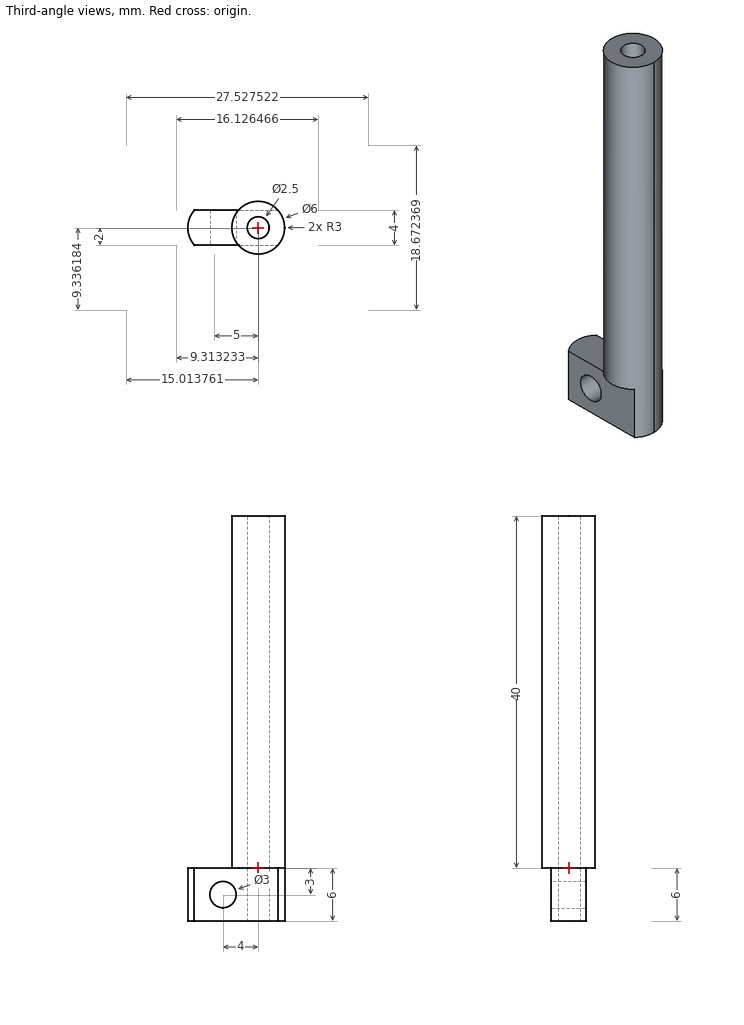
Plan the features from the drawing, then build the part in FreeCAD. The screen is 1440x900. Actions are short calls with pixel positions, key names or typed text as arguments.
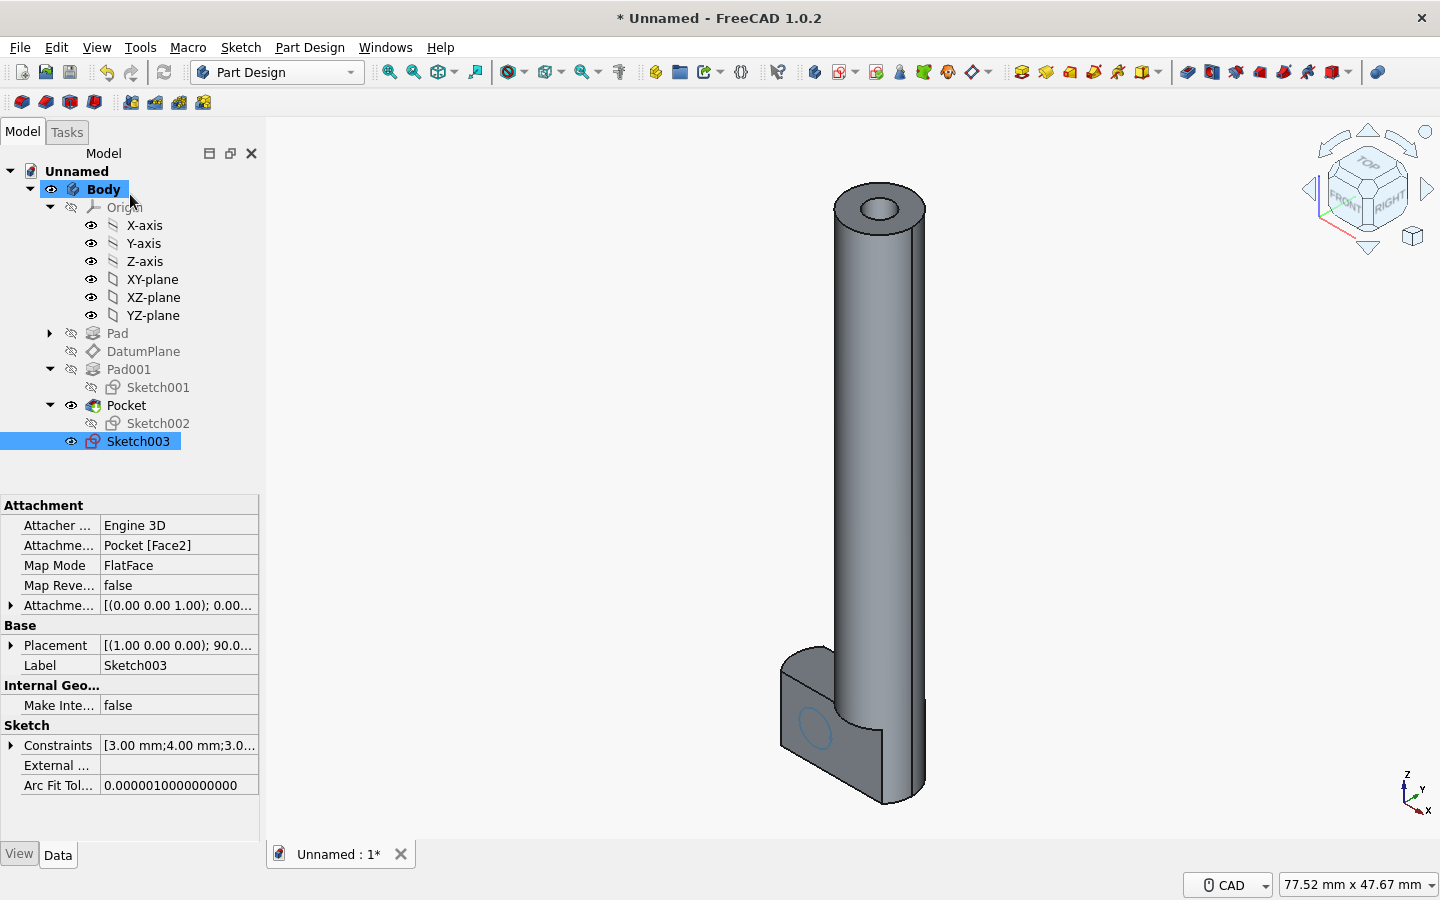
click(1188, 72)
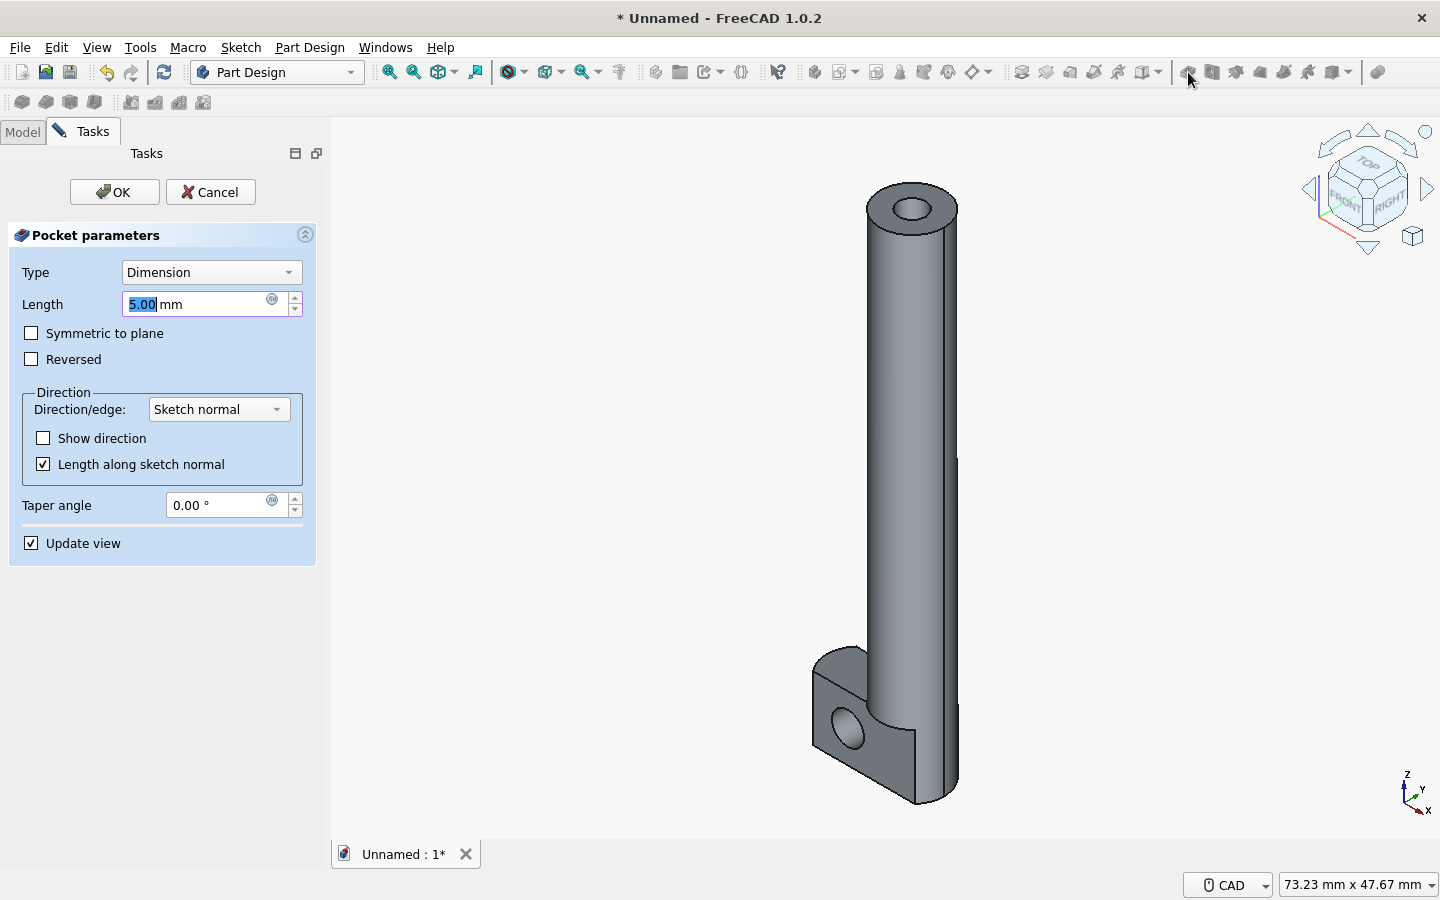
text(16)
key(Tab)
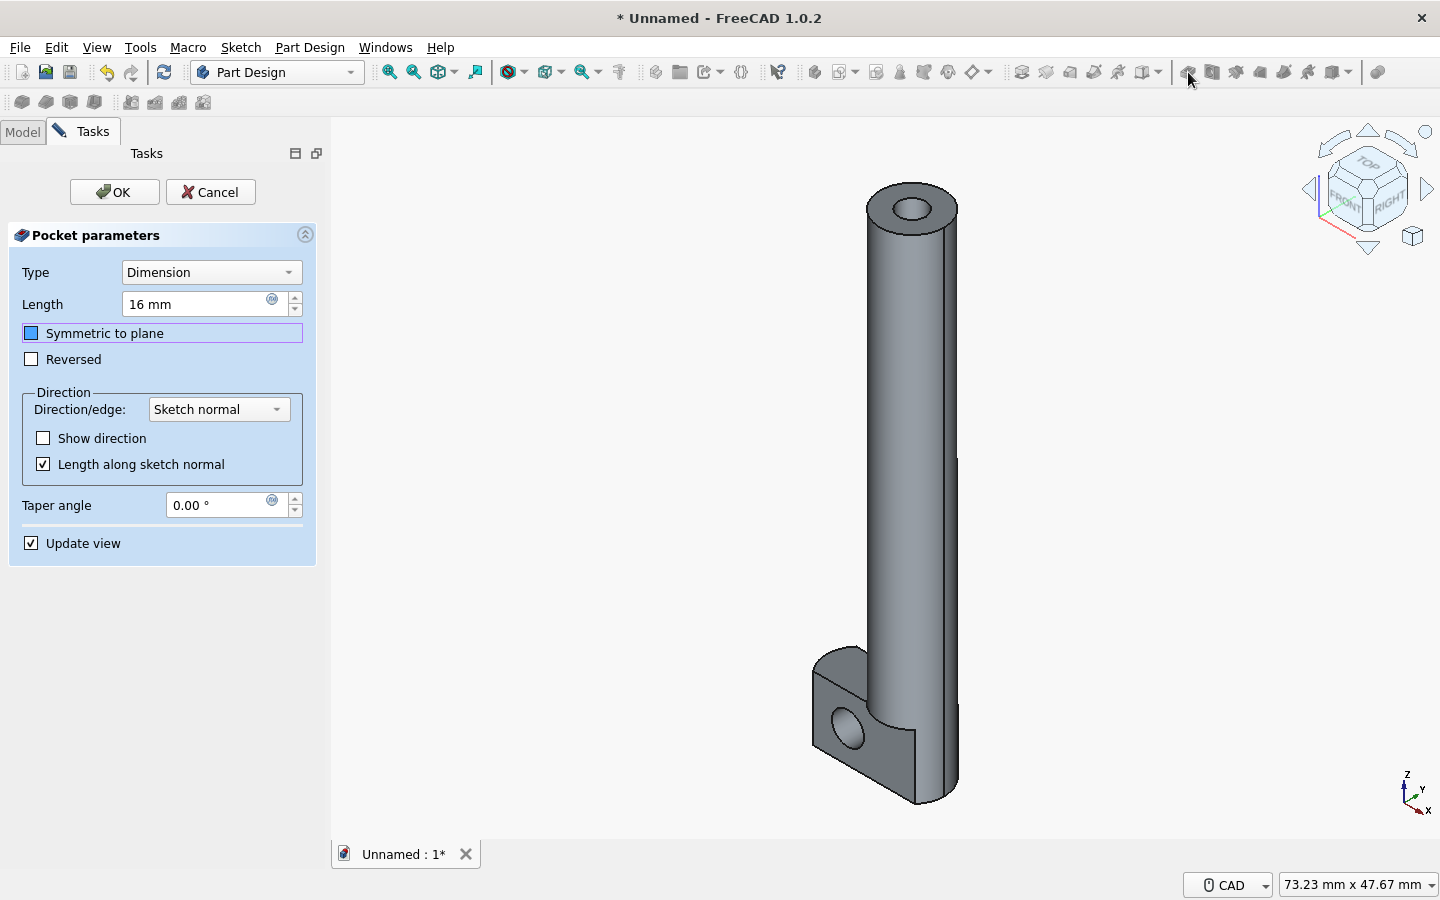
click(115, 192)